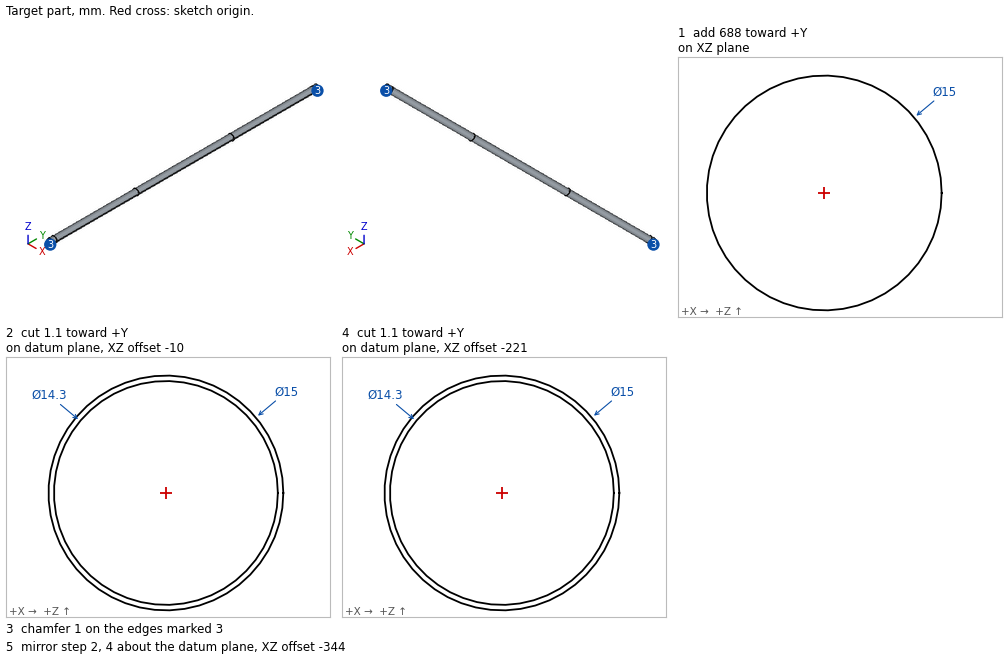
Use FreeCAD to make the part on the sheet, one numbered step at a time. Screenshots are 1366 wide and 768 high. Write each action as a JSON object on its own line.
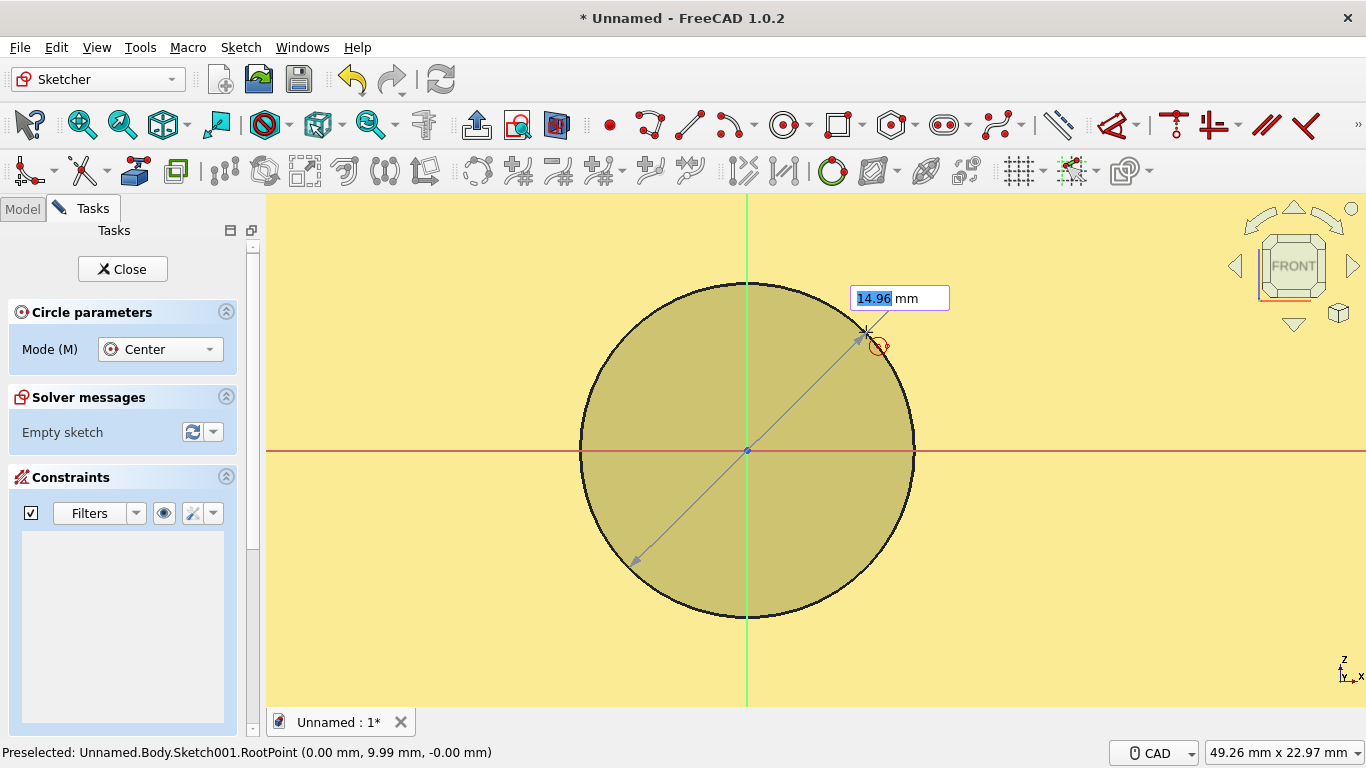
{"action": "type", "text": "15"}
{"action": "key", "text": "Return"}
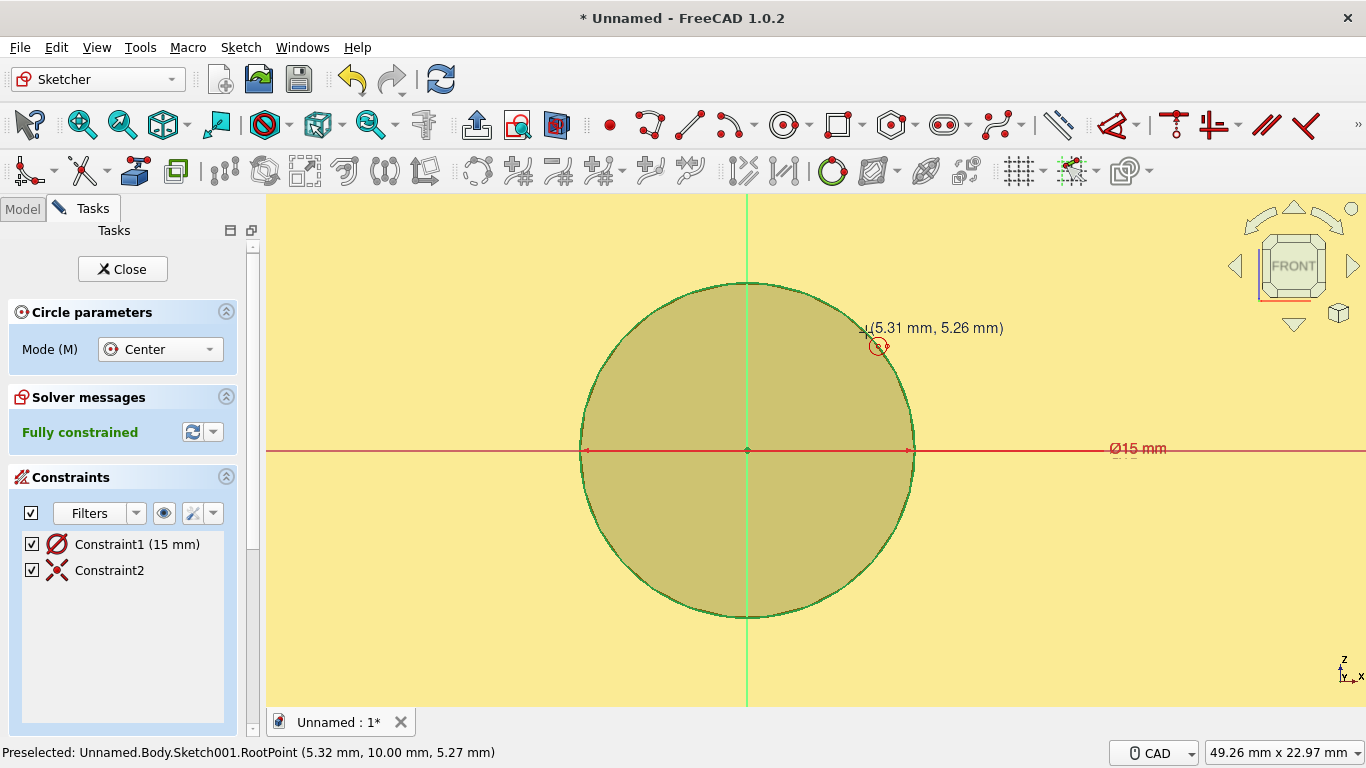
{"action": "left_click", "coordinate": [747, 451]}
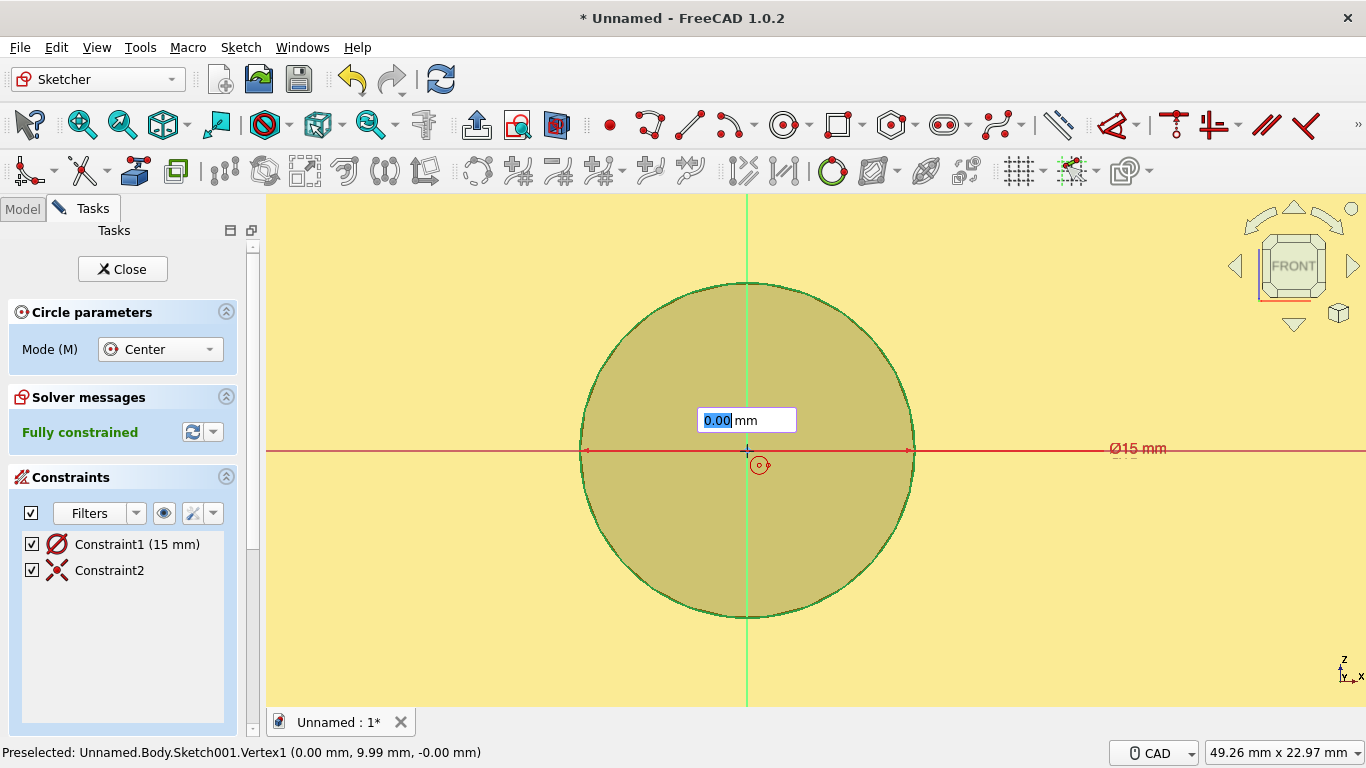
{"action": "scroll", "coordinate": [802, 301], "scroll_direction": "up", "scroll_amount": 4}
{"action": "mouse_move", "coordinate": [801, 300]}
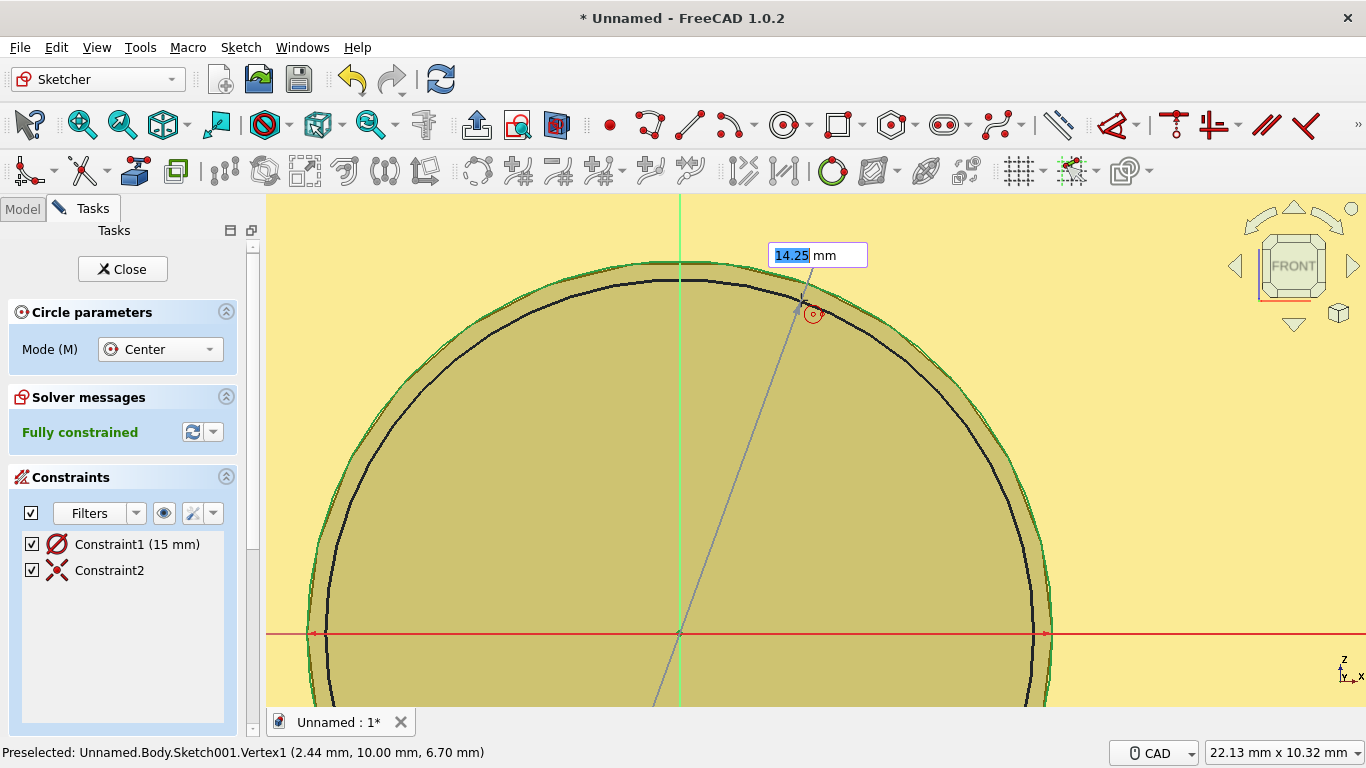
{"action": "type", "text": "14.3"}
{"action": "key", "text": "Return"}
{"action": "key", "text": "Escape"}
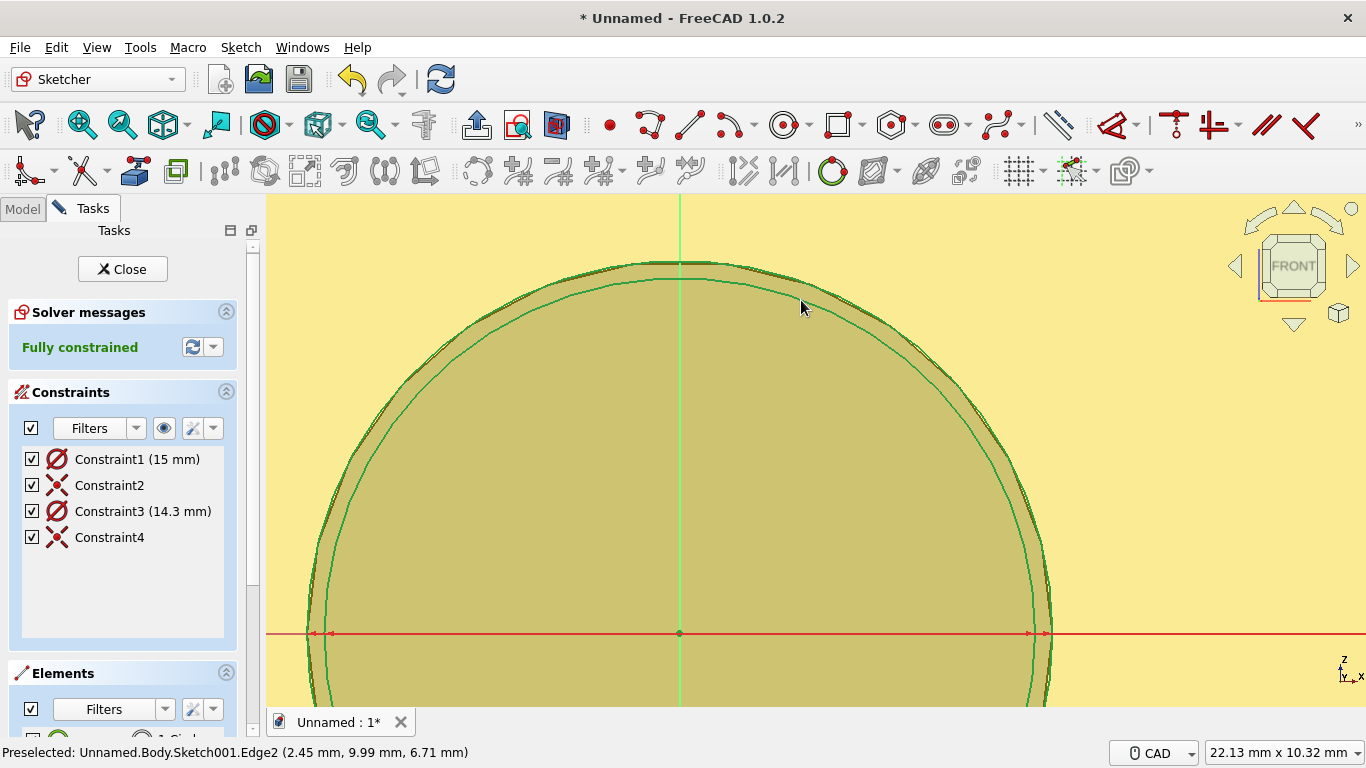
{"action": "left_click", "coordinate": [123, 269]}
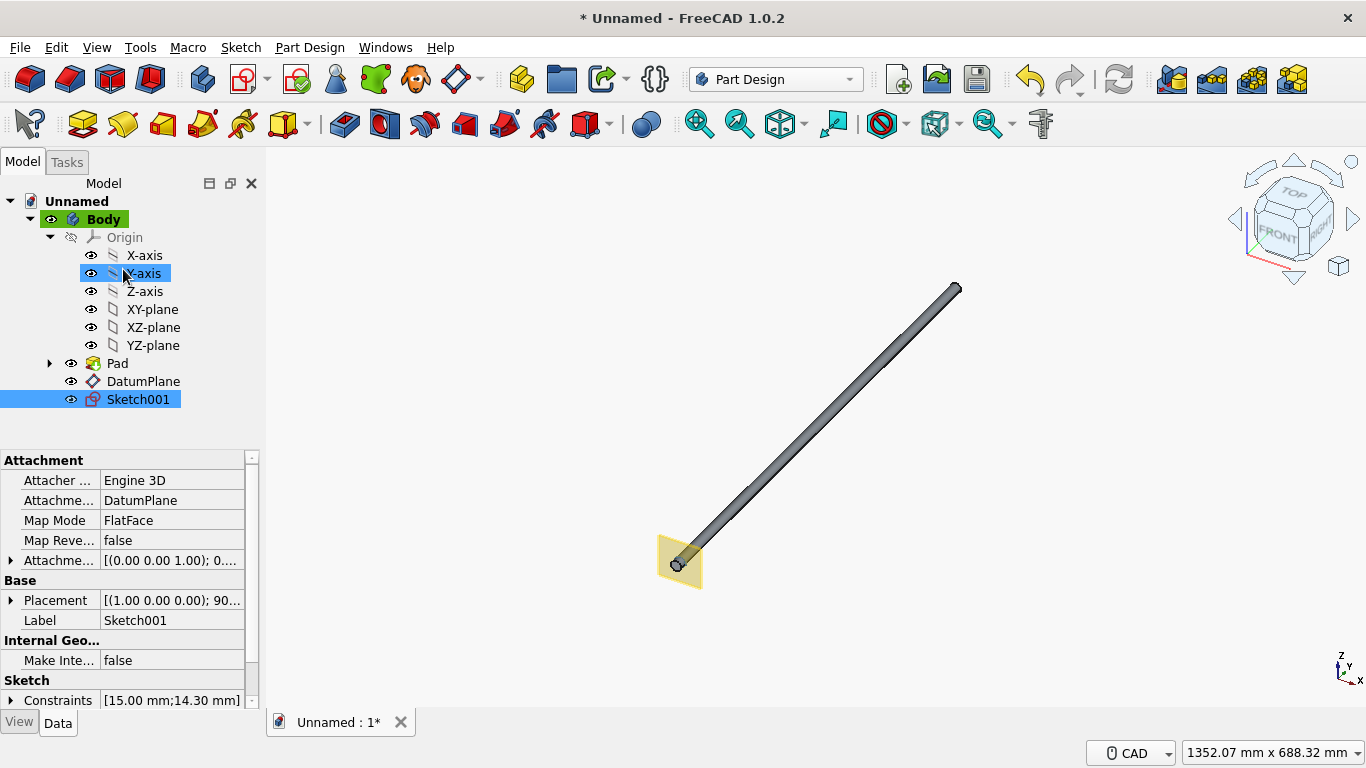
{"action": "left_click", "coordinate": [346, 124]}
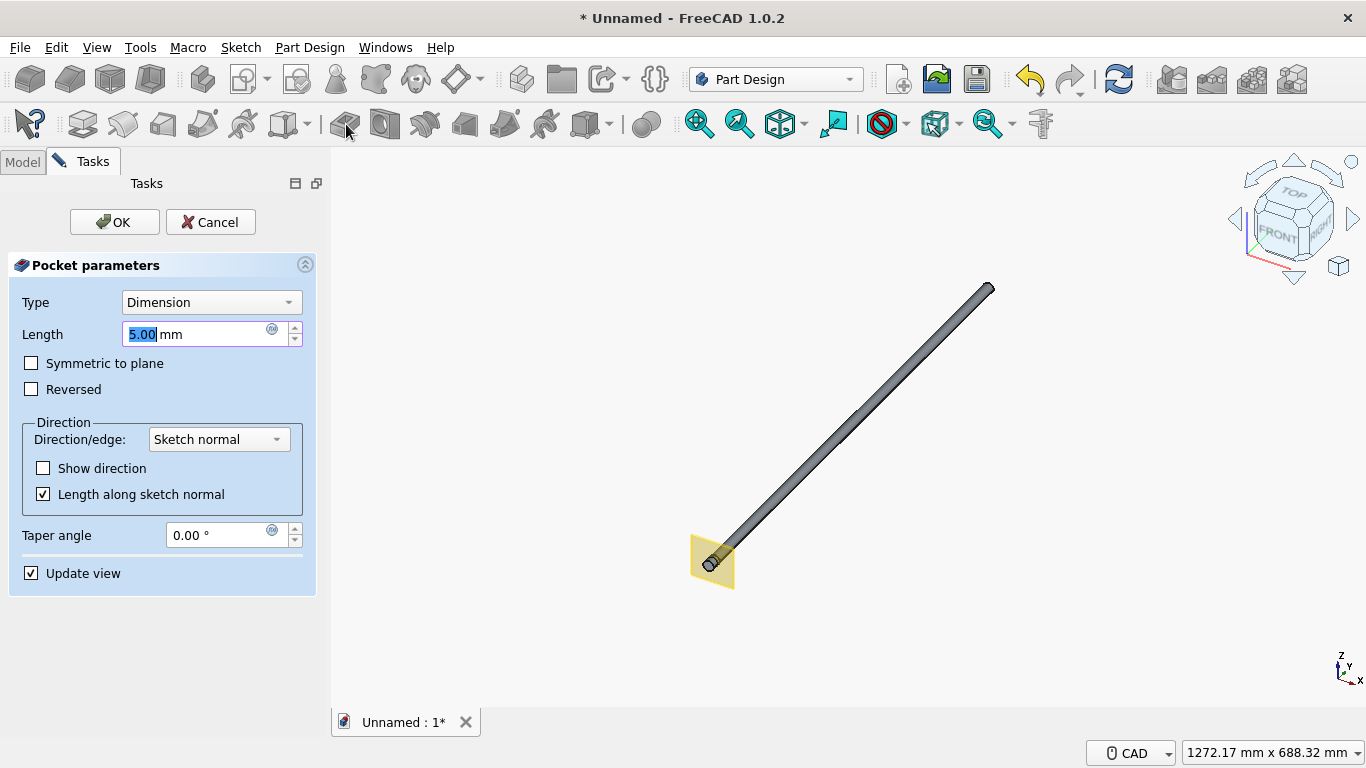
{"action": "type", "text": "1.1"}
{"action": "key", "text": "Tab"}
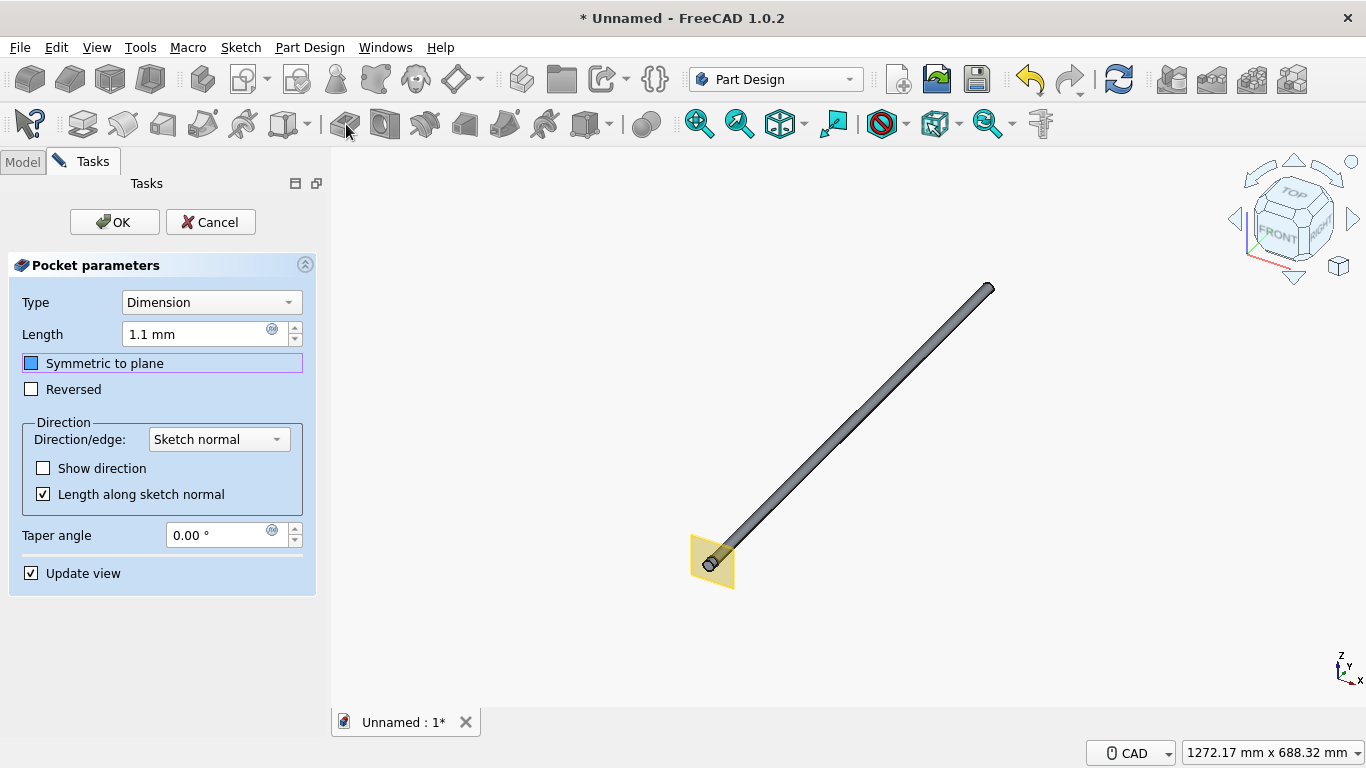
{"action": "left_click", "coordinate": [115, 222]}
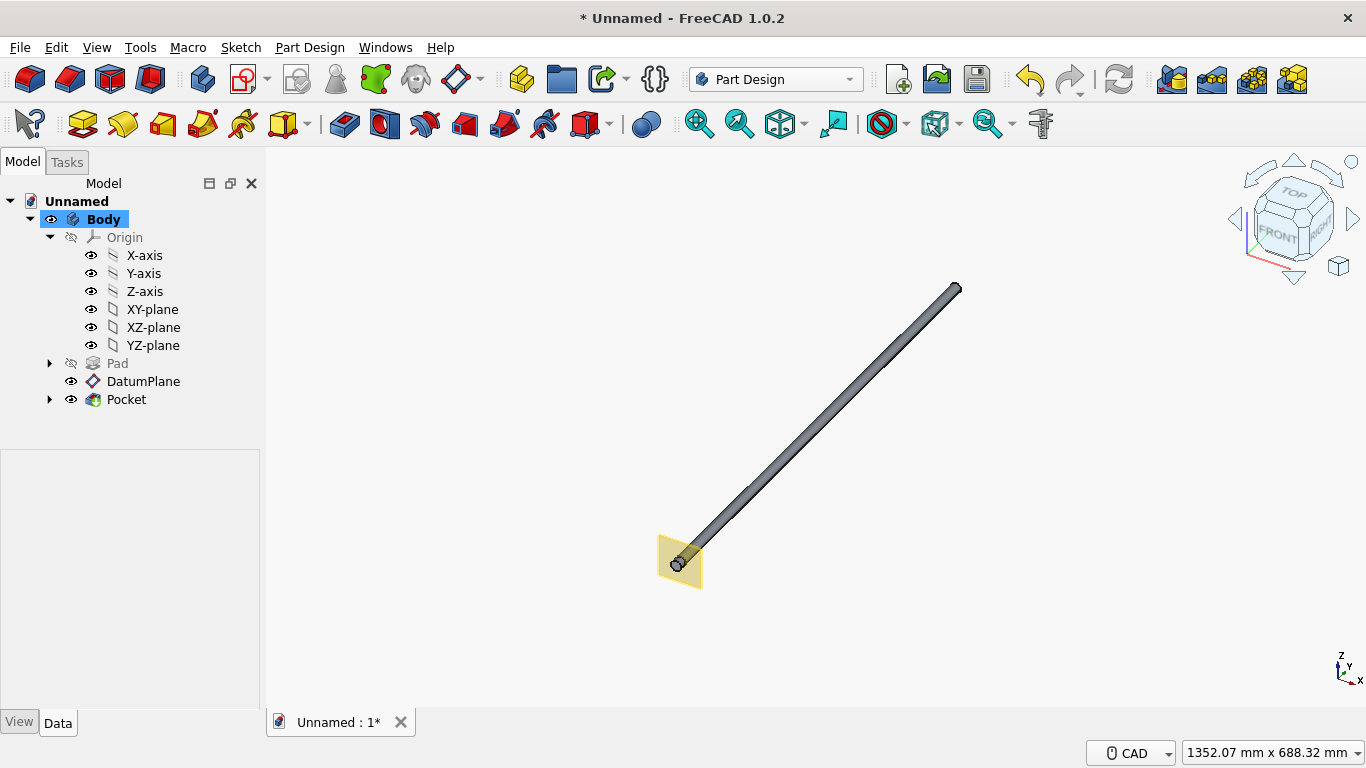
{"action": "left_click", "coordinate": [116, 381]}
{"action": "key", "text": "space"}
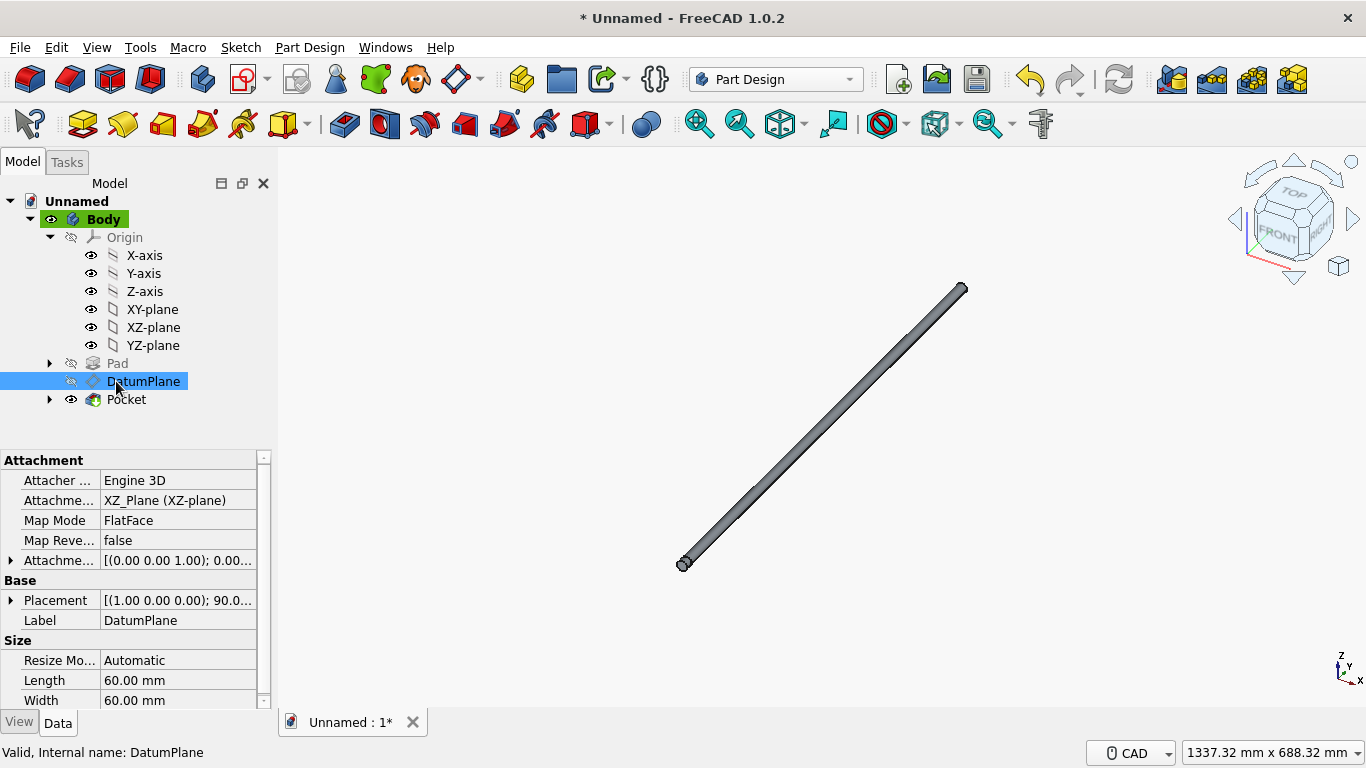
{"action": "left_click", "coordinate": [677, 563]}